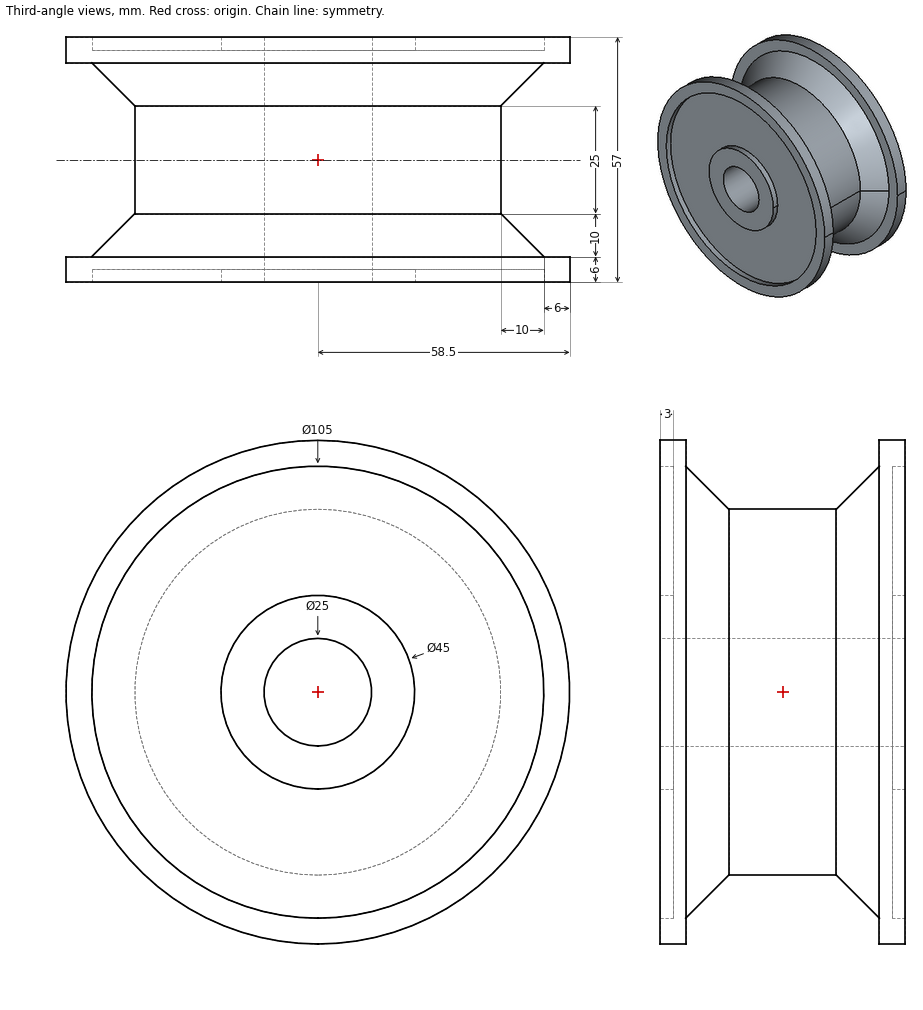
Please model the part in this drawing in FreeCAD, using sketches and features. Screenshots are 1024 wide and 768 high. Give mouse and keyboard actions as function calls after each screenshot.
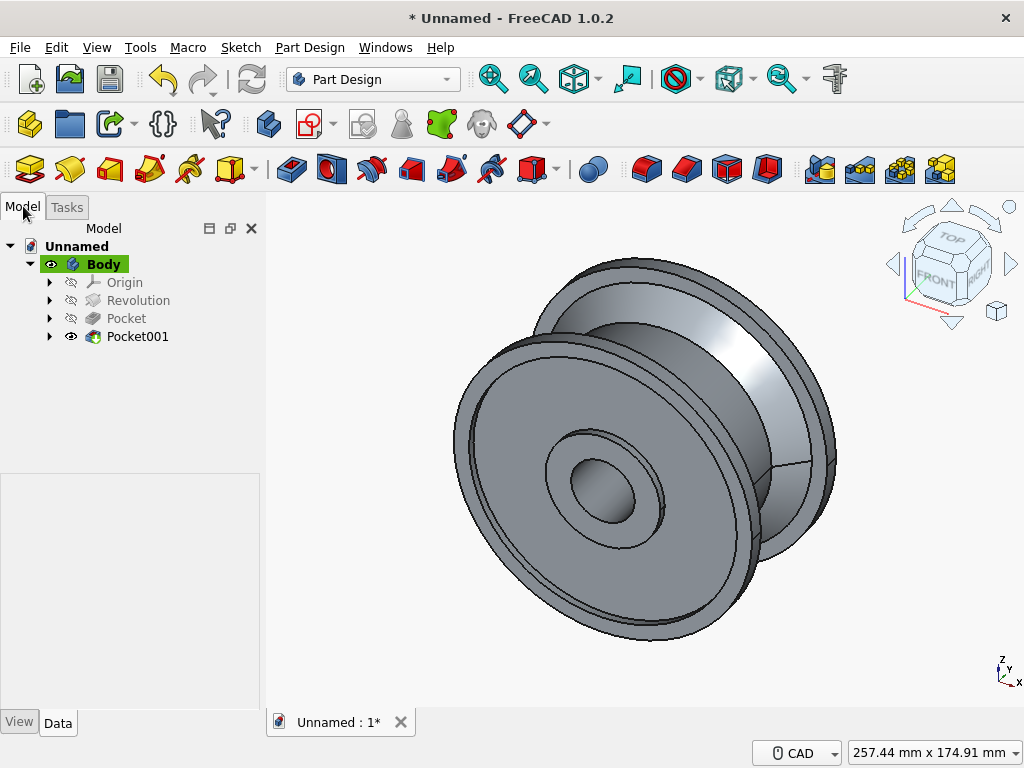
click(116, 336)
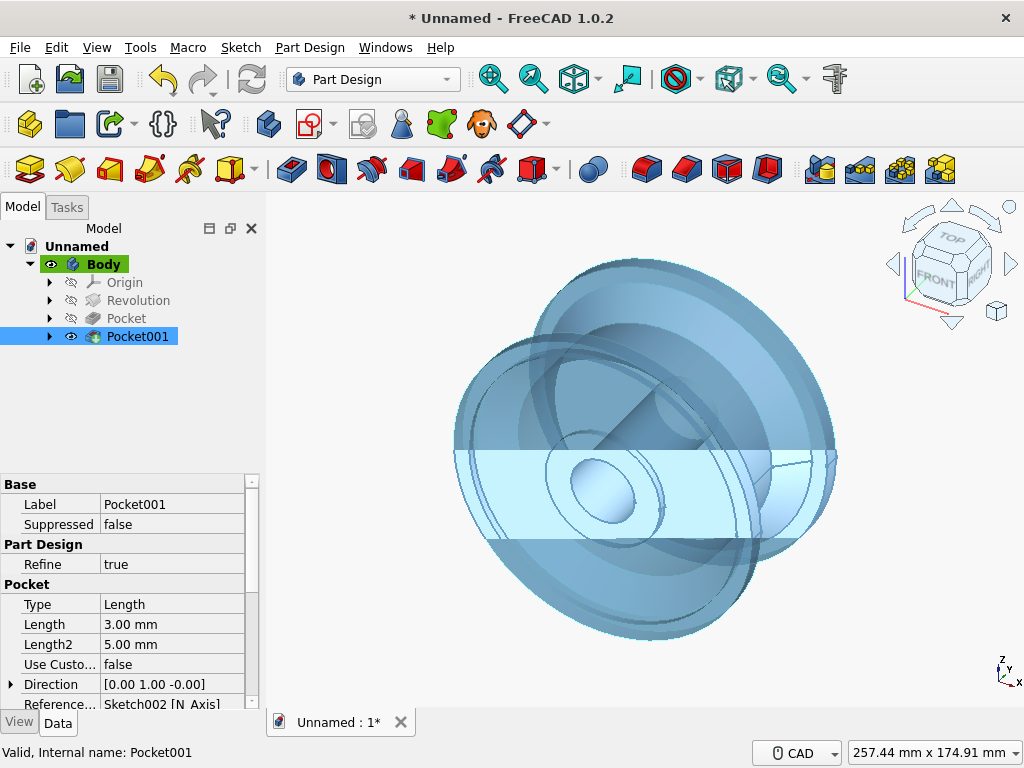
click(820, 170)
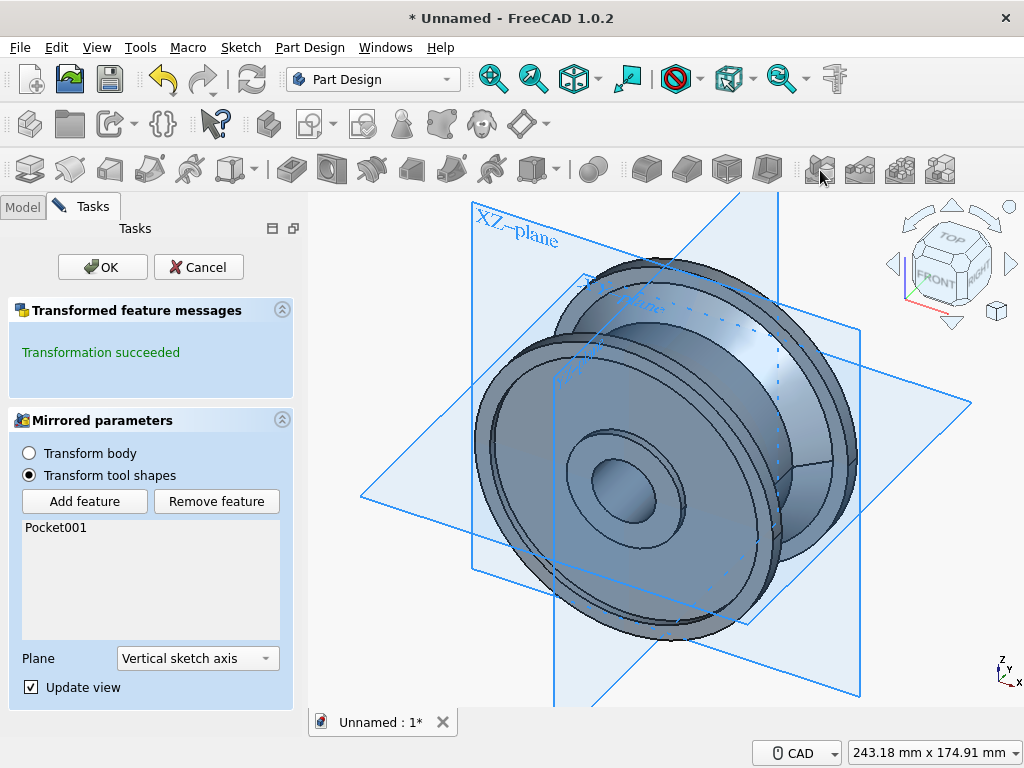
click(198, 658)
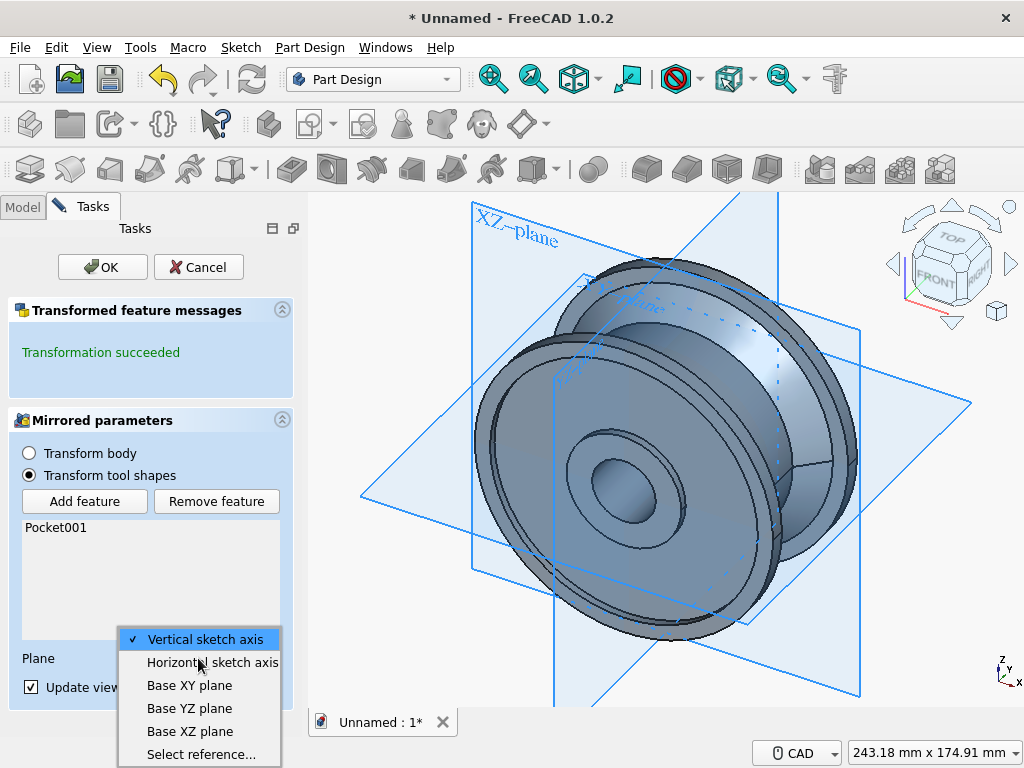
click(198, 732)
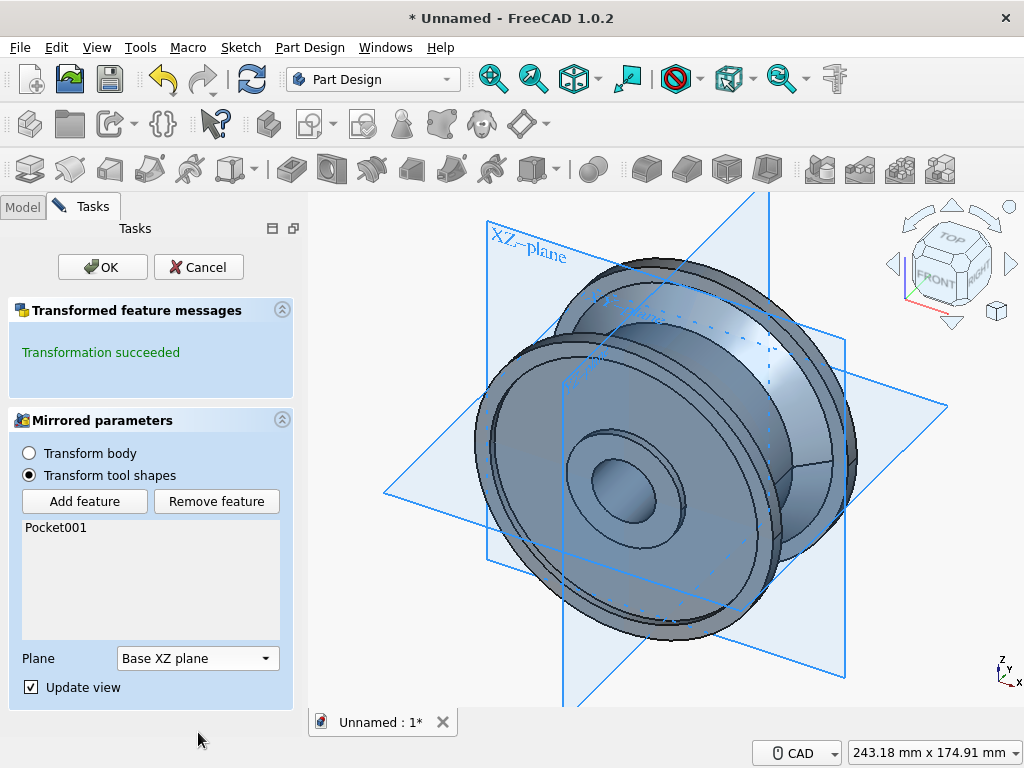
click(103, 267)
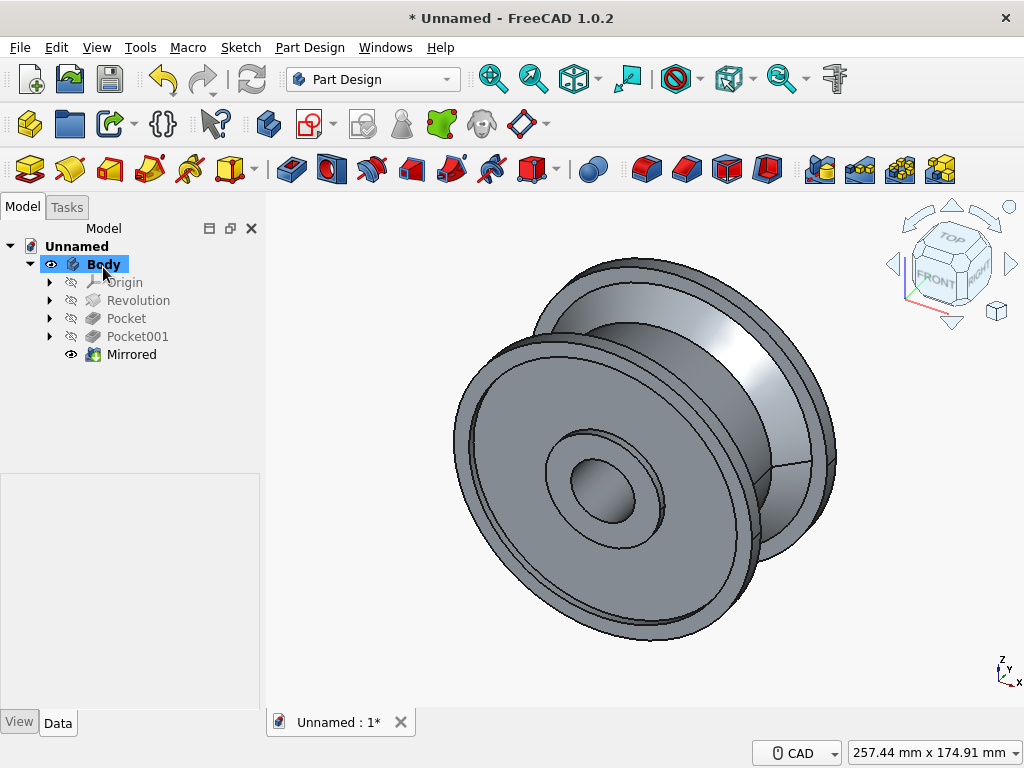
key(0)